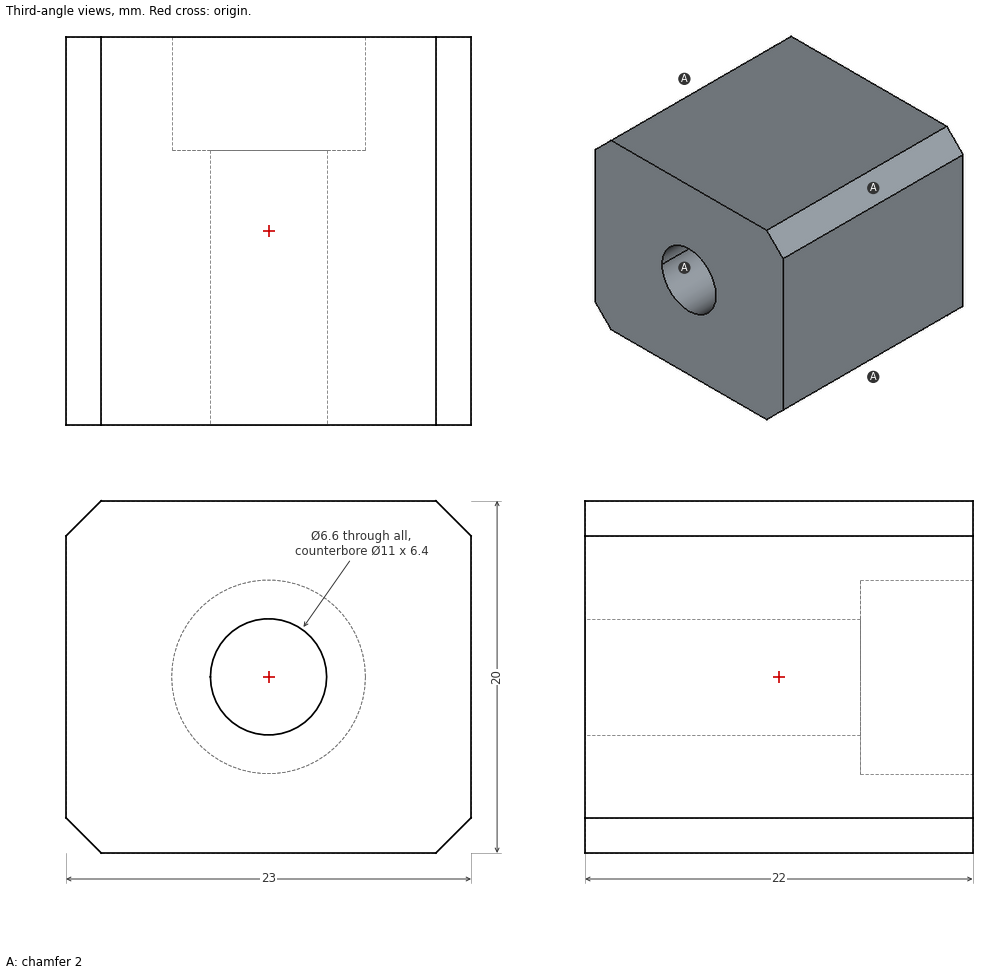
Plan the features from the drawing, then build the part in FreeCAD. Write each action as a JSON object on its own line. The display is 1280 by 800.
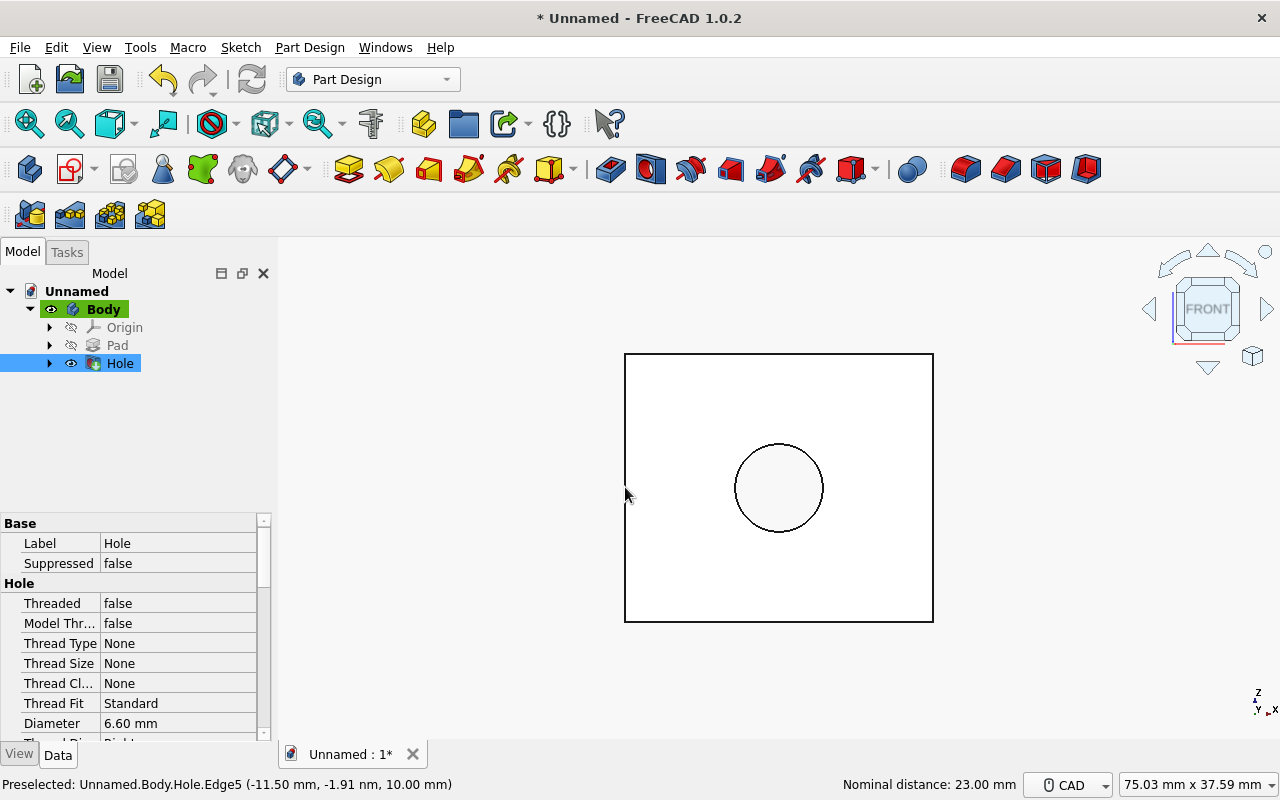
{"action": "key", "text": "3"}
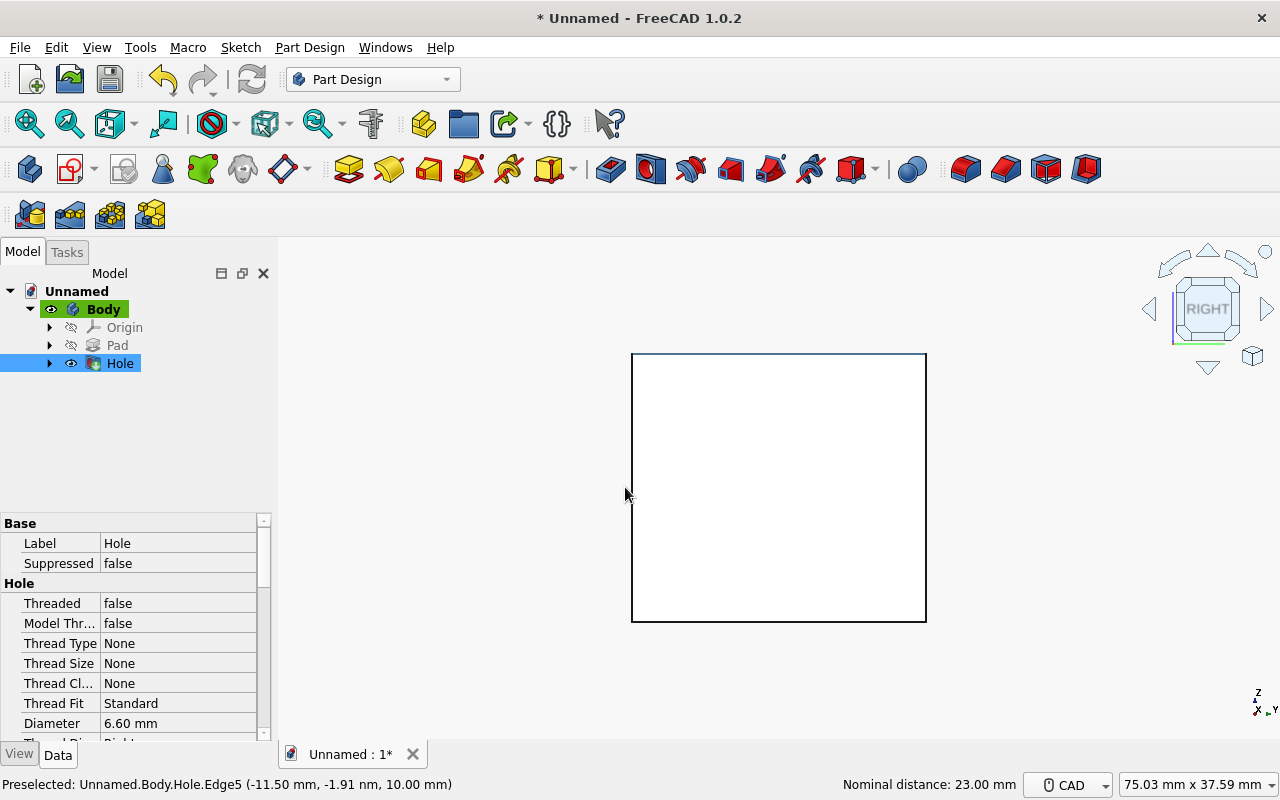
{"action": "left_click", "coordinate": [779, 621], "text": "ctrl"}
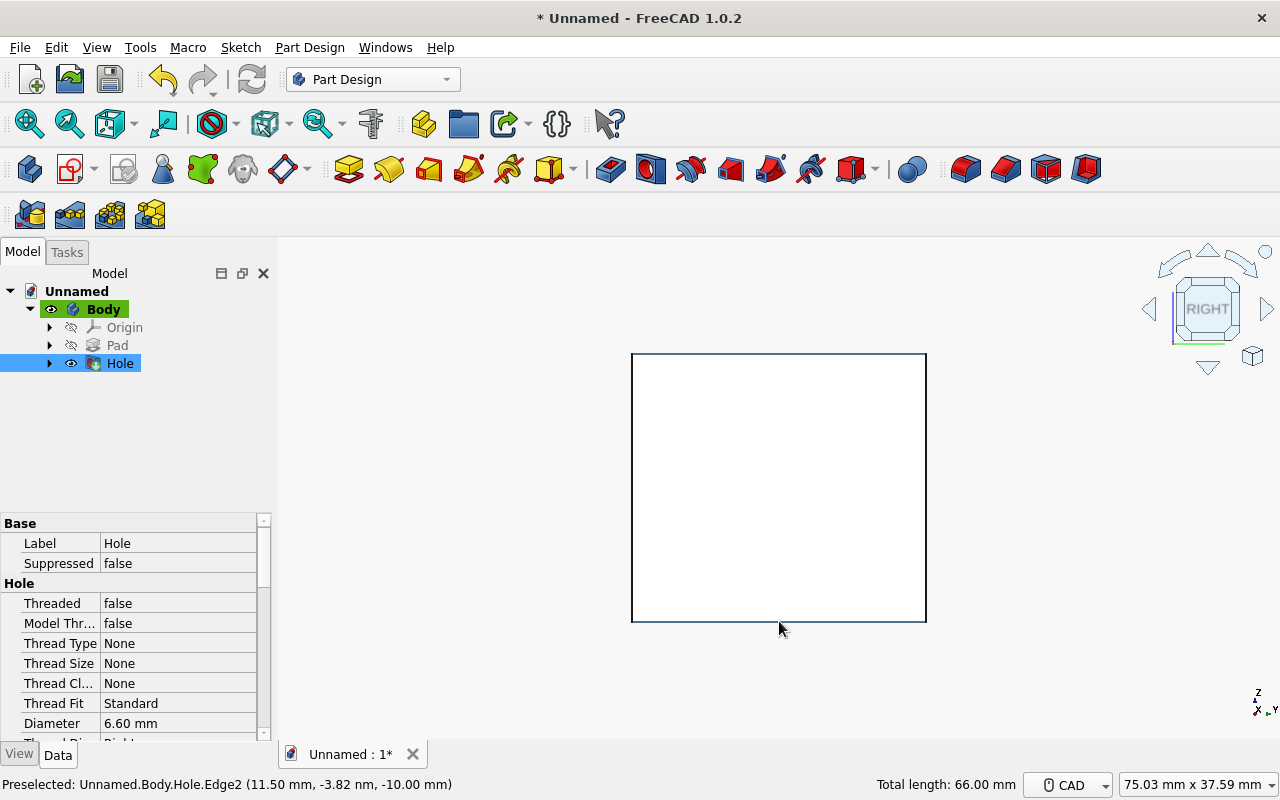
{"action": "key", "text": "5"}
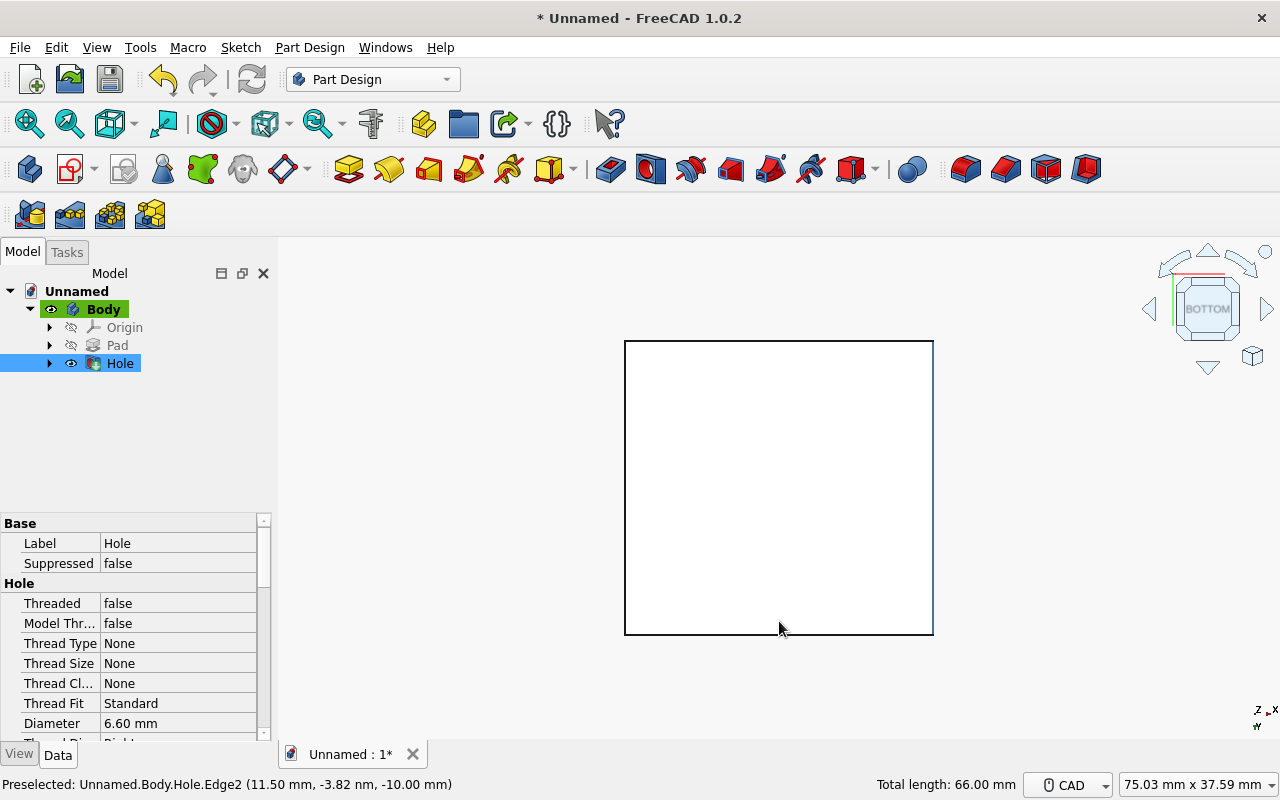
{"action": "left_click", "coordinate": [625, 487], "text": "ctrl"}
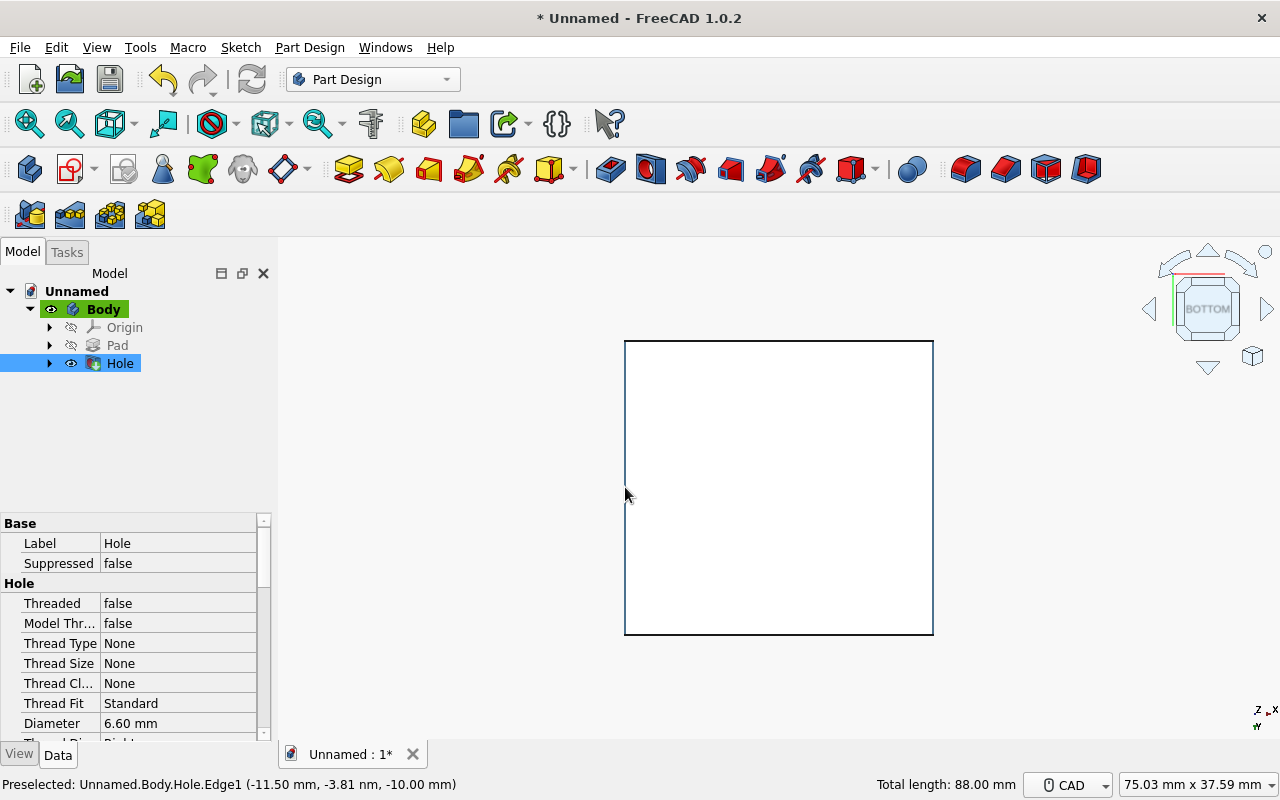
{"action": "left_click", "coordinate": [1006, 170]}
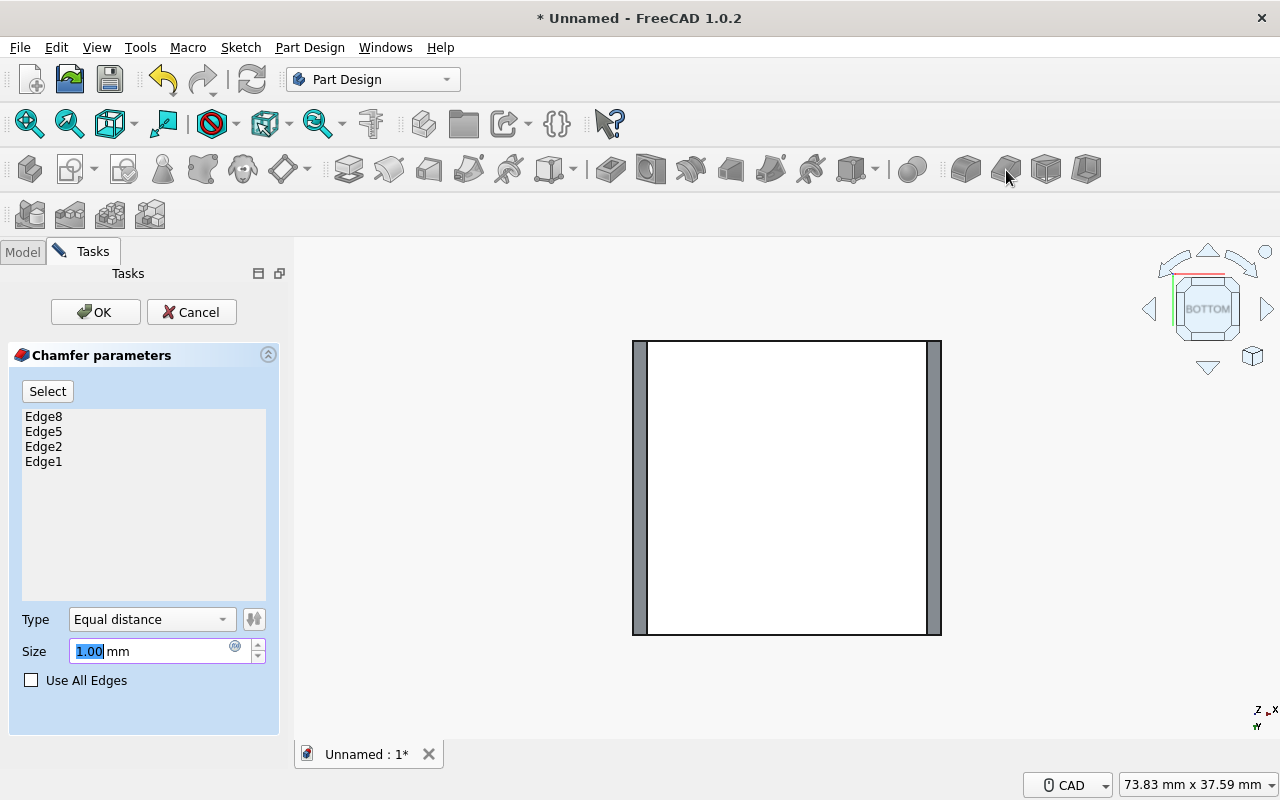
{"action": "type", "text": "2"}
{"action": "key", "text": "Tab"}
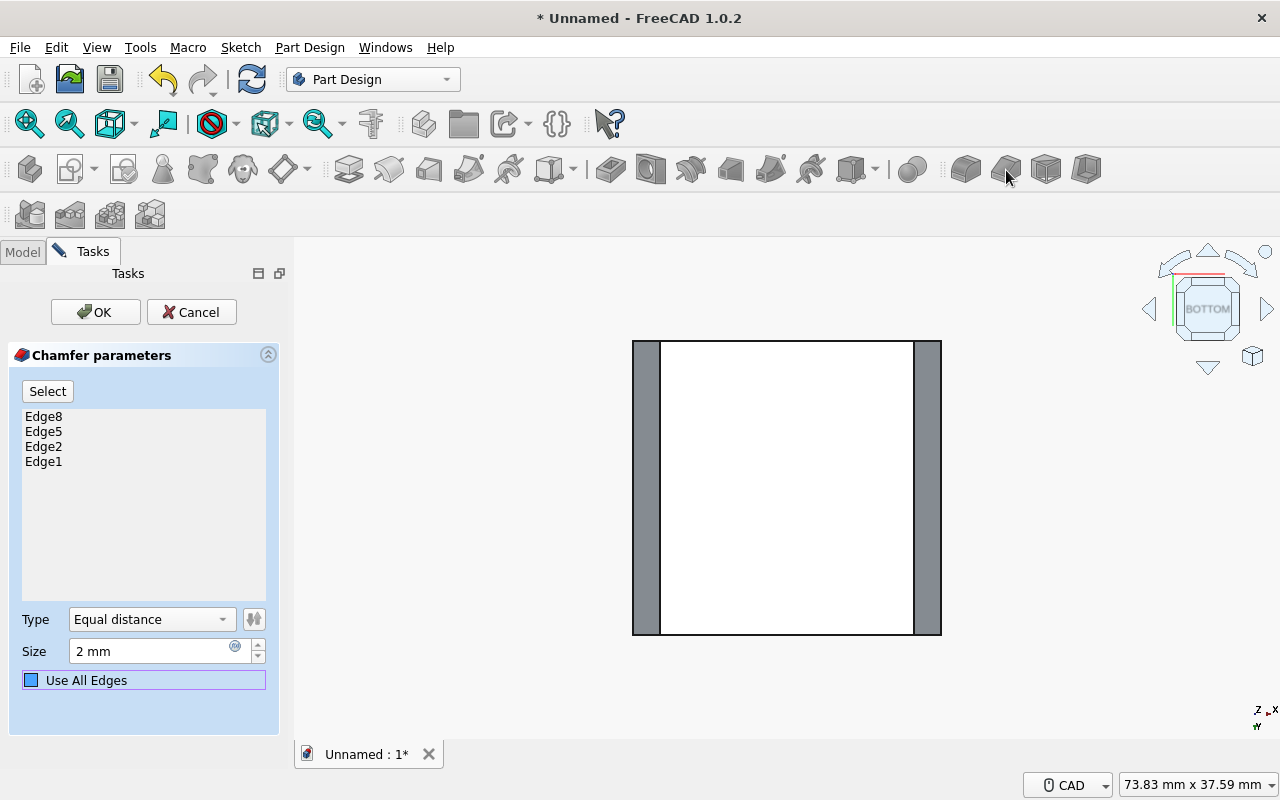
{"action": "left_click", "coordinate": [96, 312]}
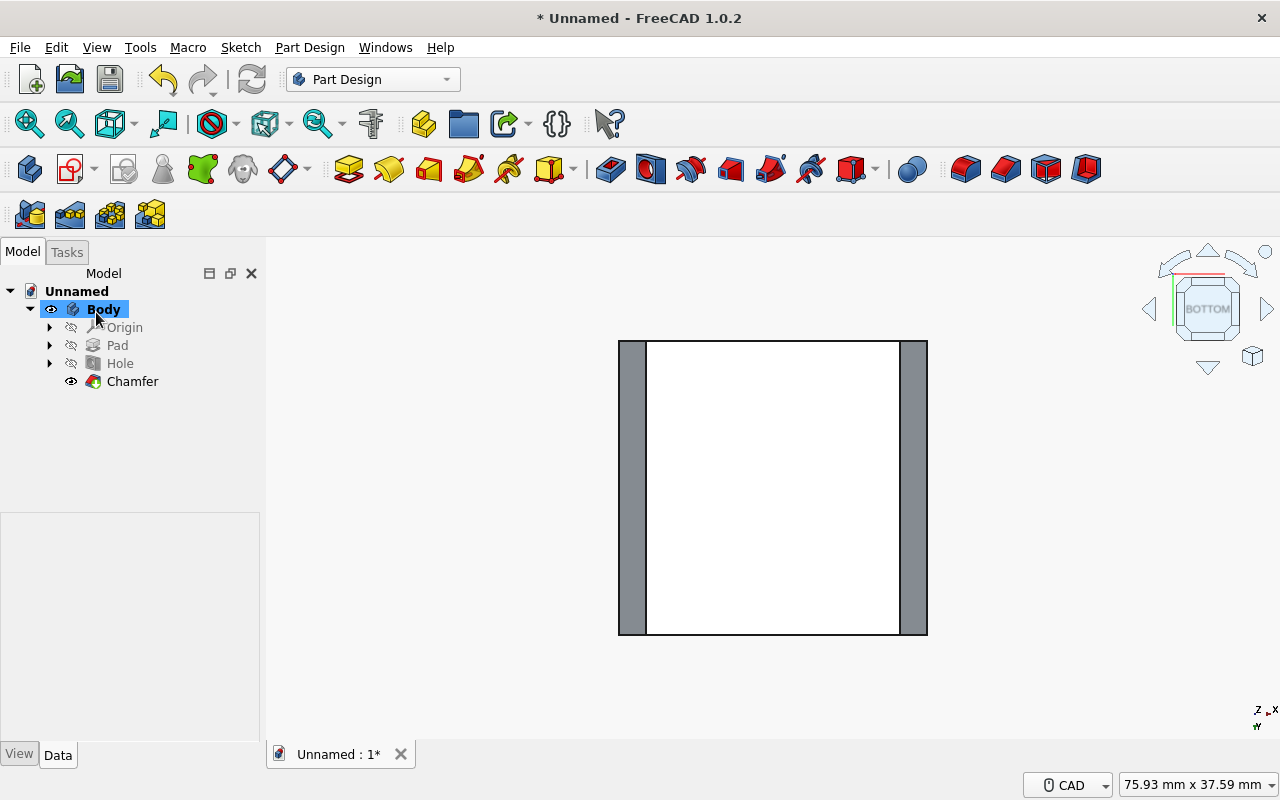
{"action": "key", "text": "0"}